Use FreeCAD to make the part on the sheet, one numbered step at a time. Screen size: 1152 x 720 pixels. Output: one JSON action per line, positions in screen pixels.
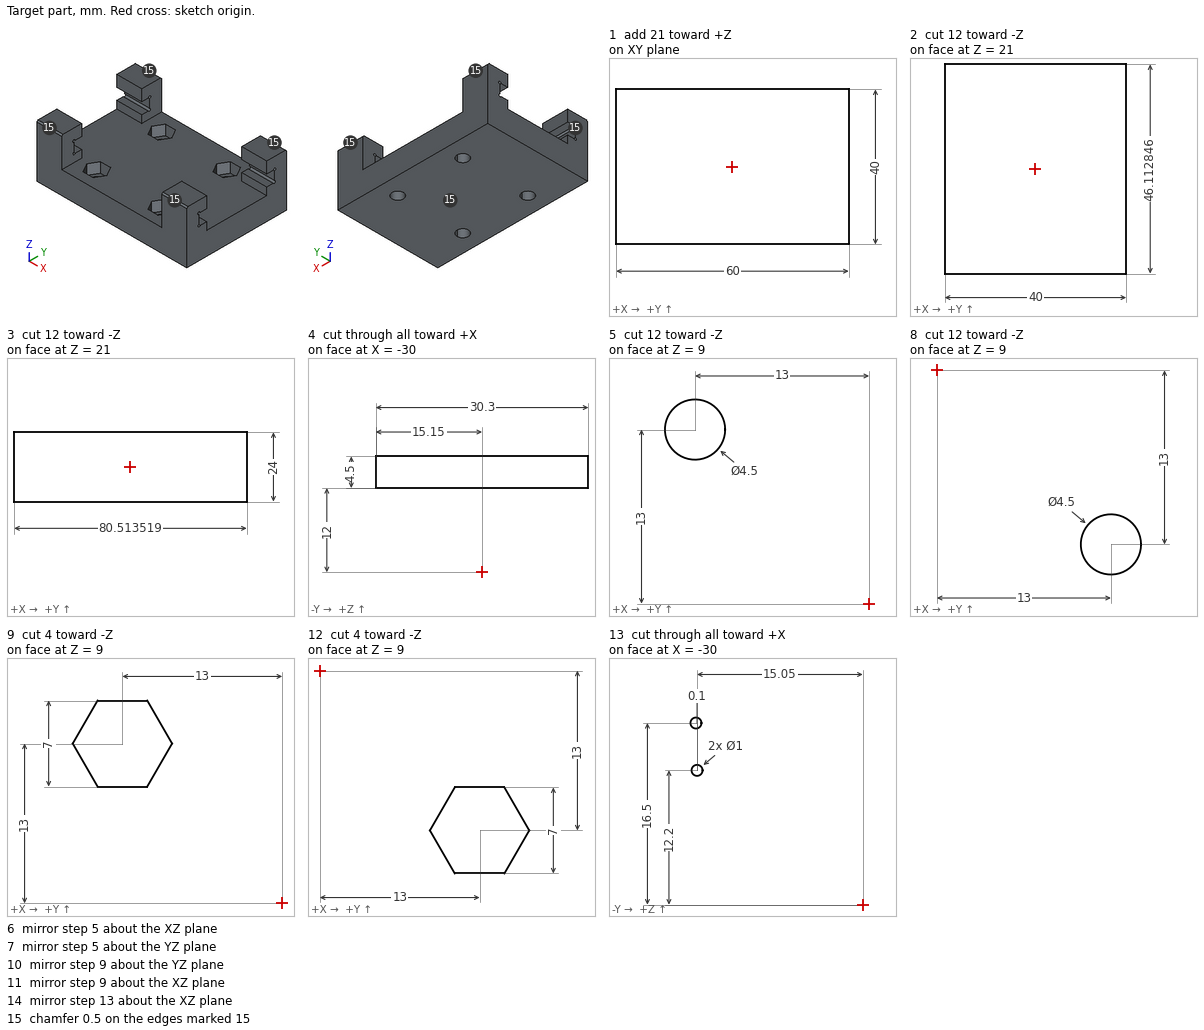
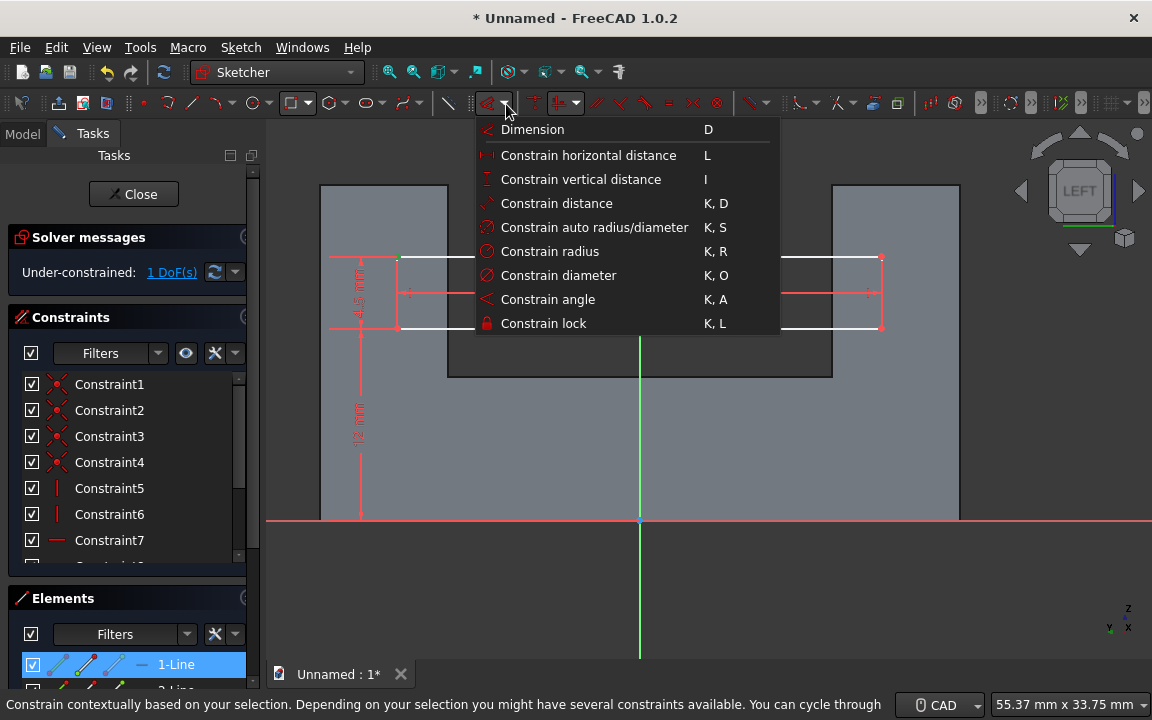
{"action": "left_click", "coordinate": [628, 155]}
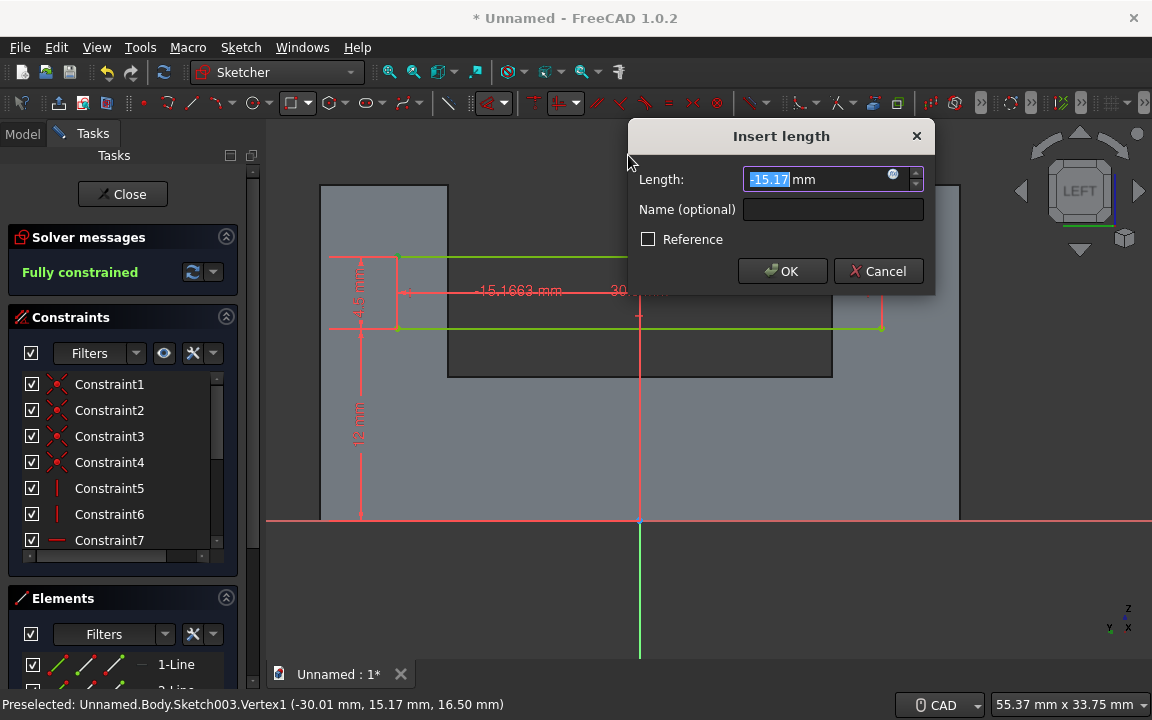
{"action": "type", "text": "-15.15"}
{"action": "key", "text": "Return"}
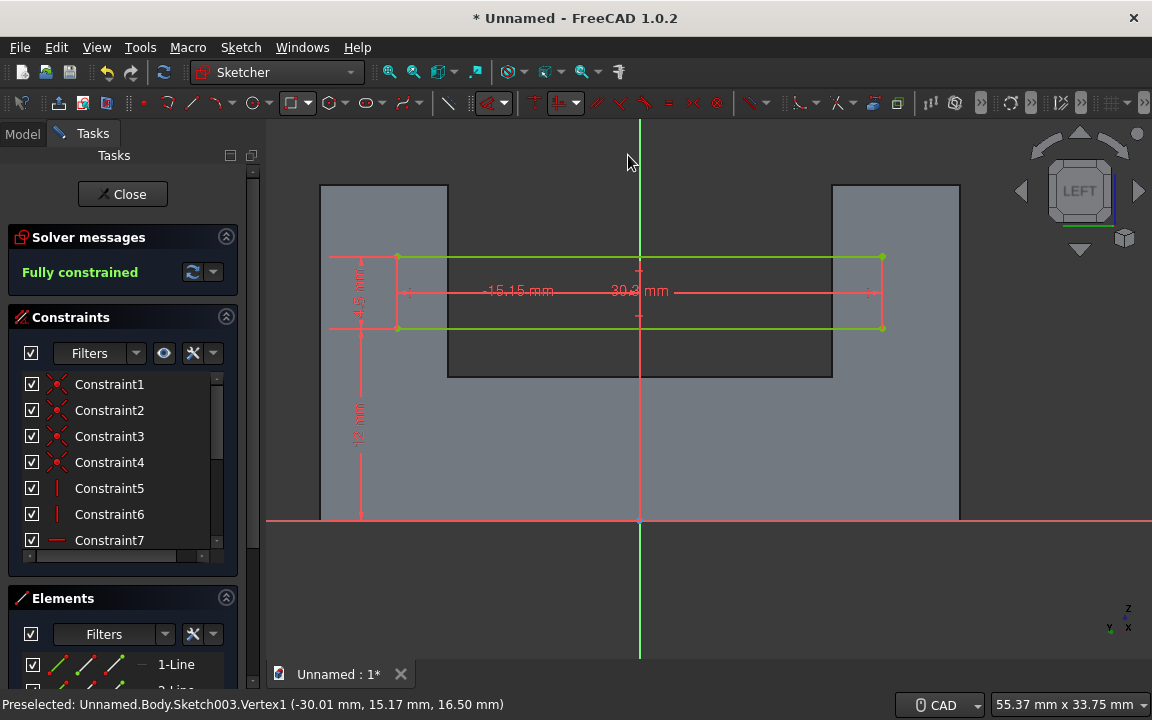
{"action": "left_click", "coordinate": [123, 194]}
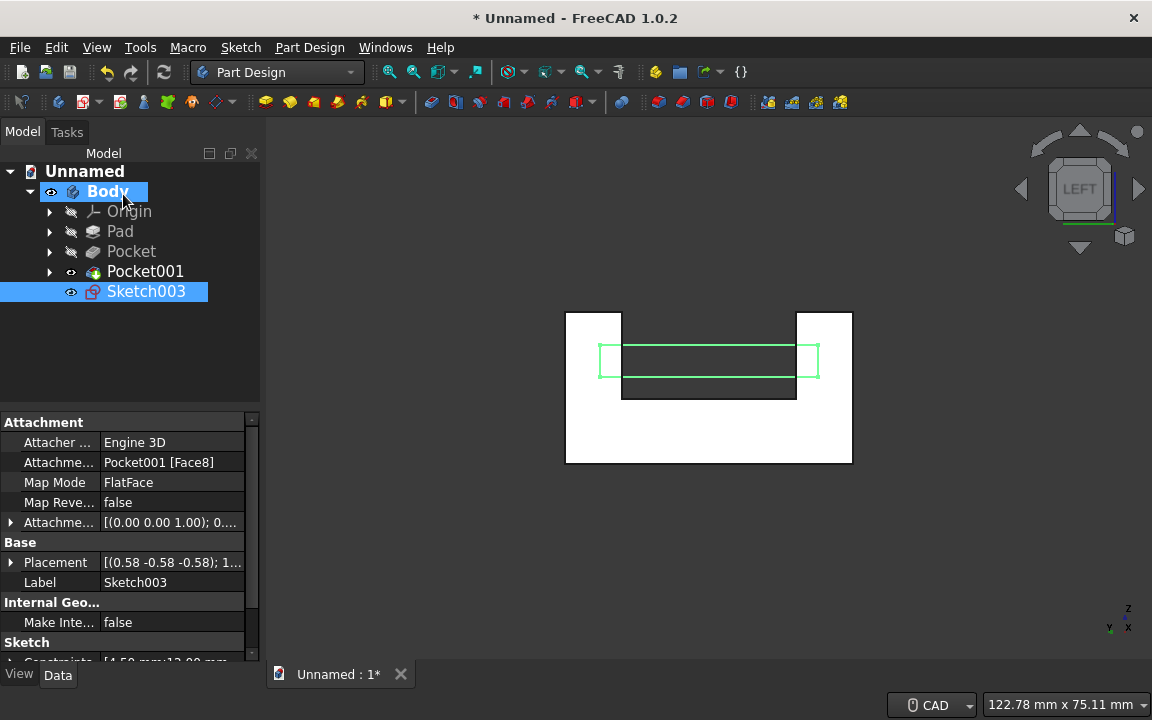
{"action": "left_click", "coordinate": [432, 102]}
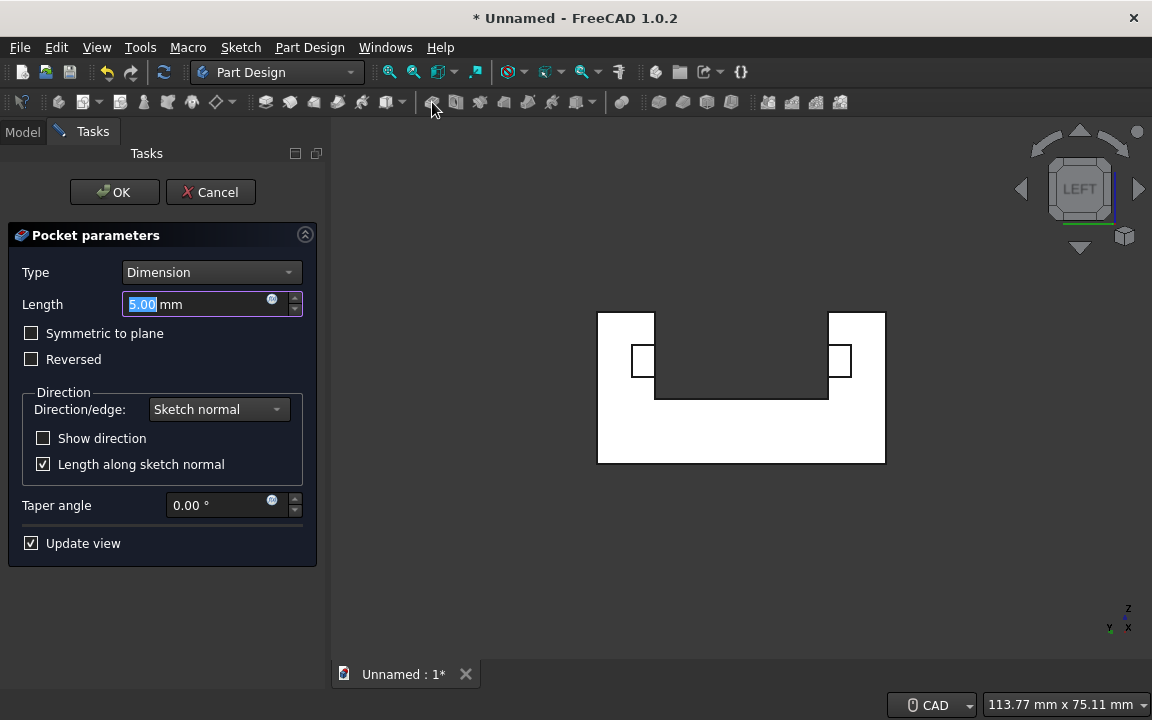
{"action": "left_click", "coordinate": [212, 272]}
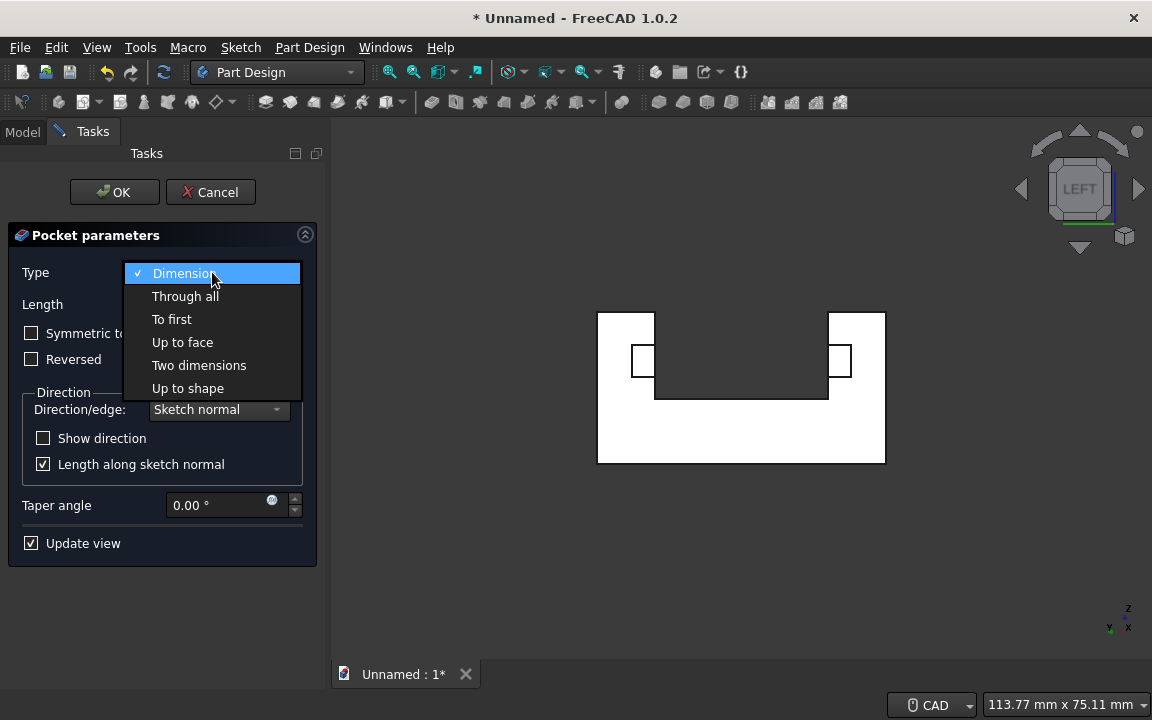
{"action": "left_click", "coordinate": [212, 296]}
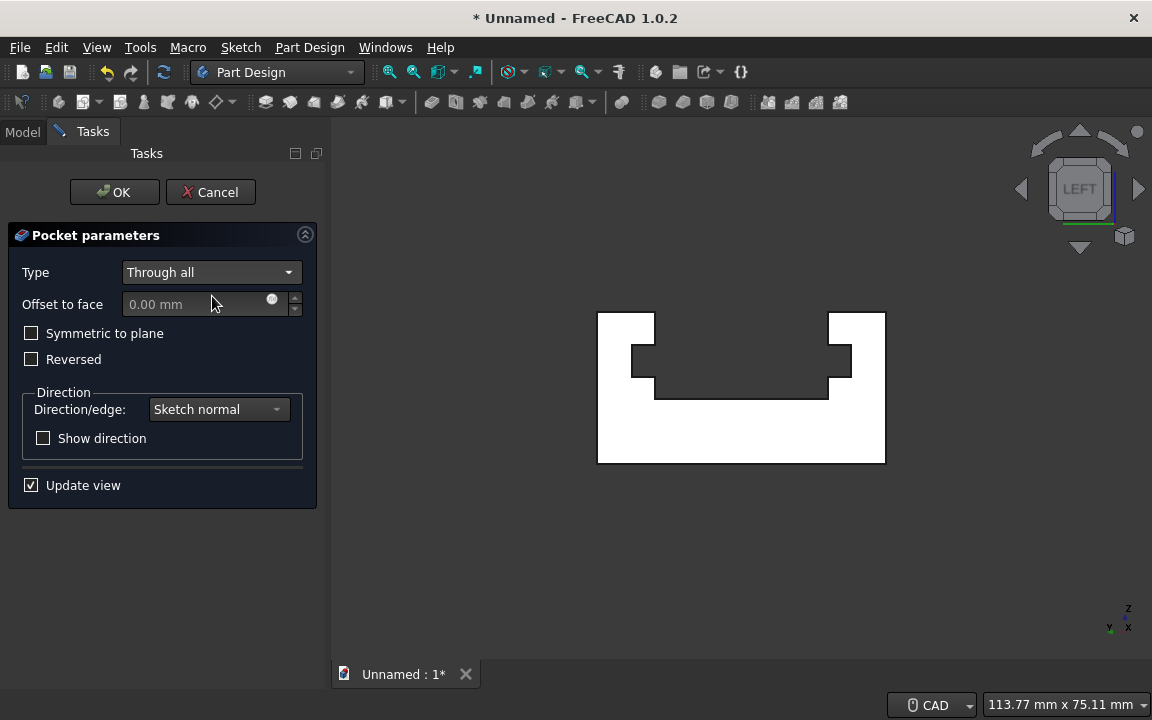
{"action": "left_click", "coordinate": [115, 192]}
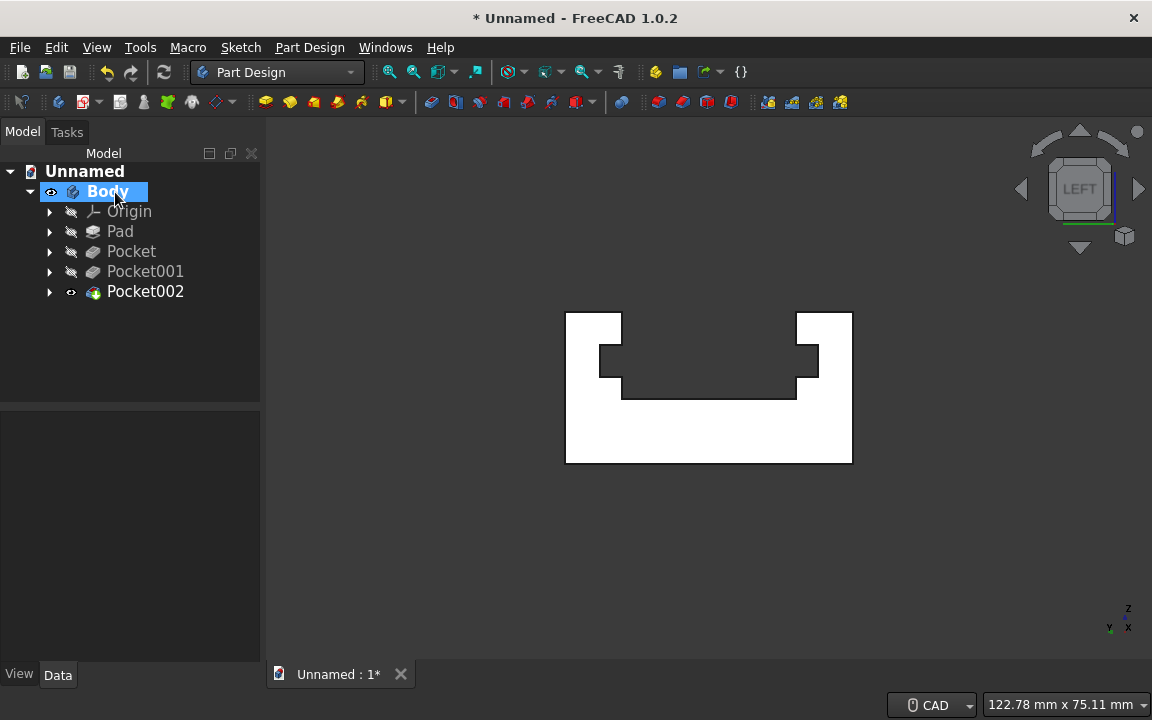
{"action": "left_click", "coordinate": [390, 72]}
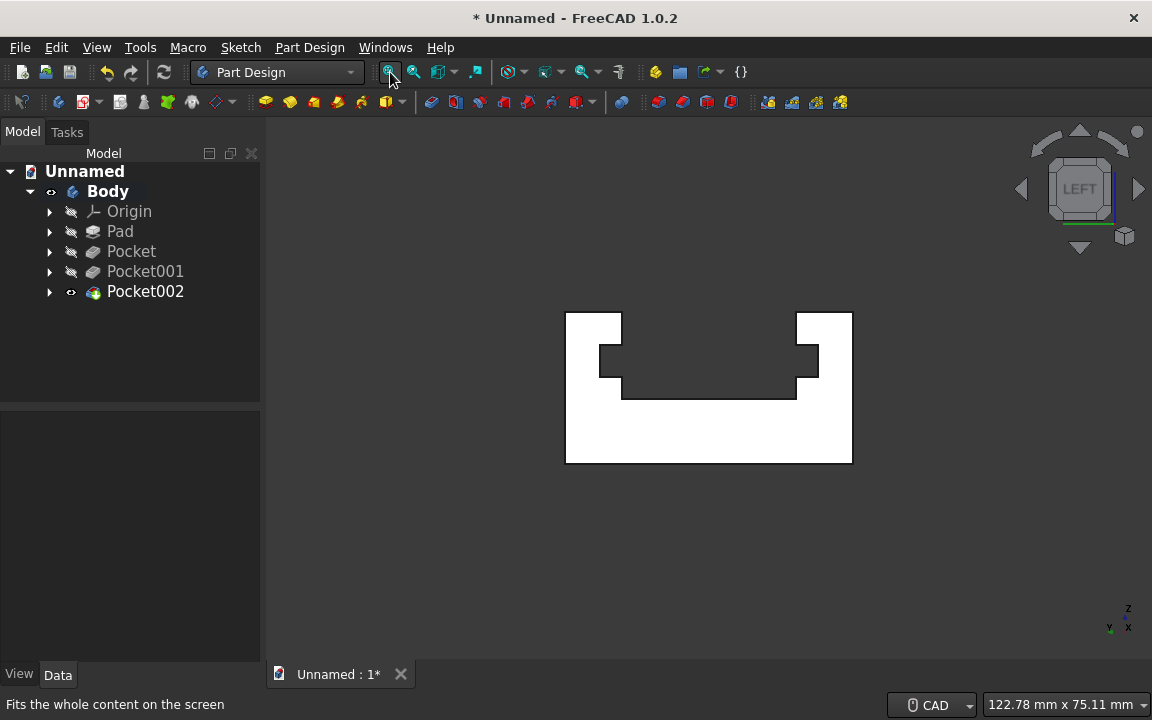
{"action": "key", "text": "0"}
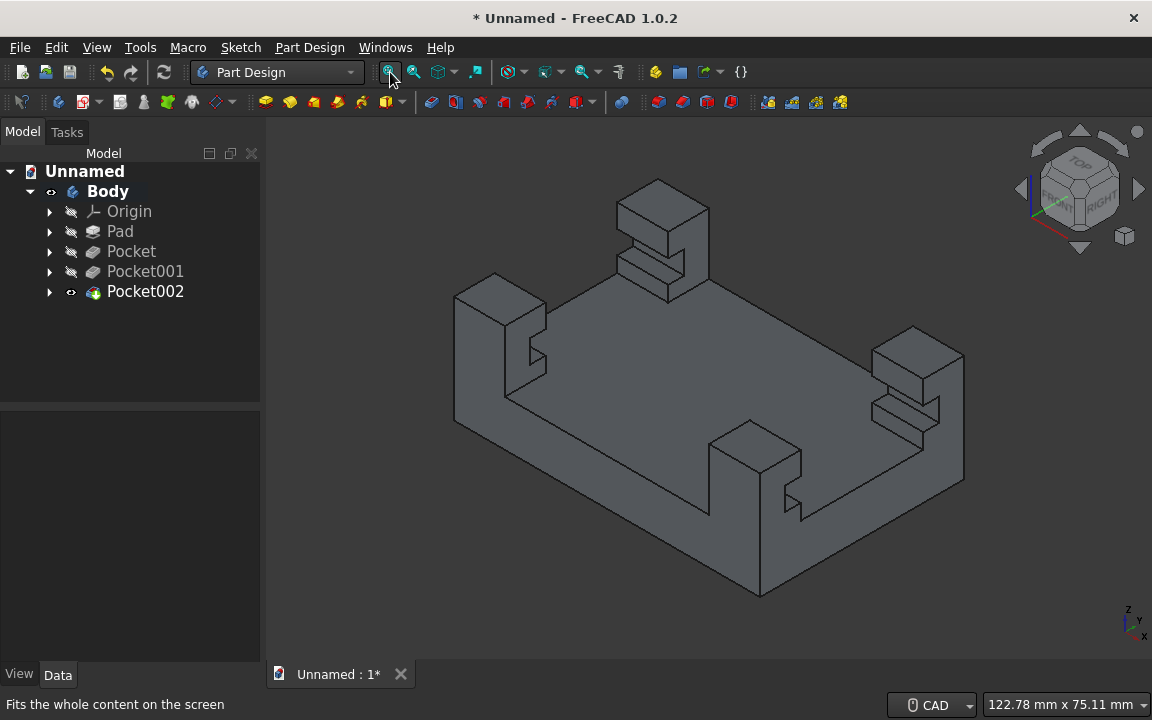
{"action": "left_click", "coordinate": [709, 396]}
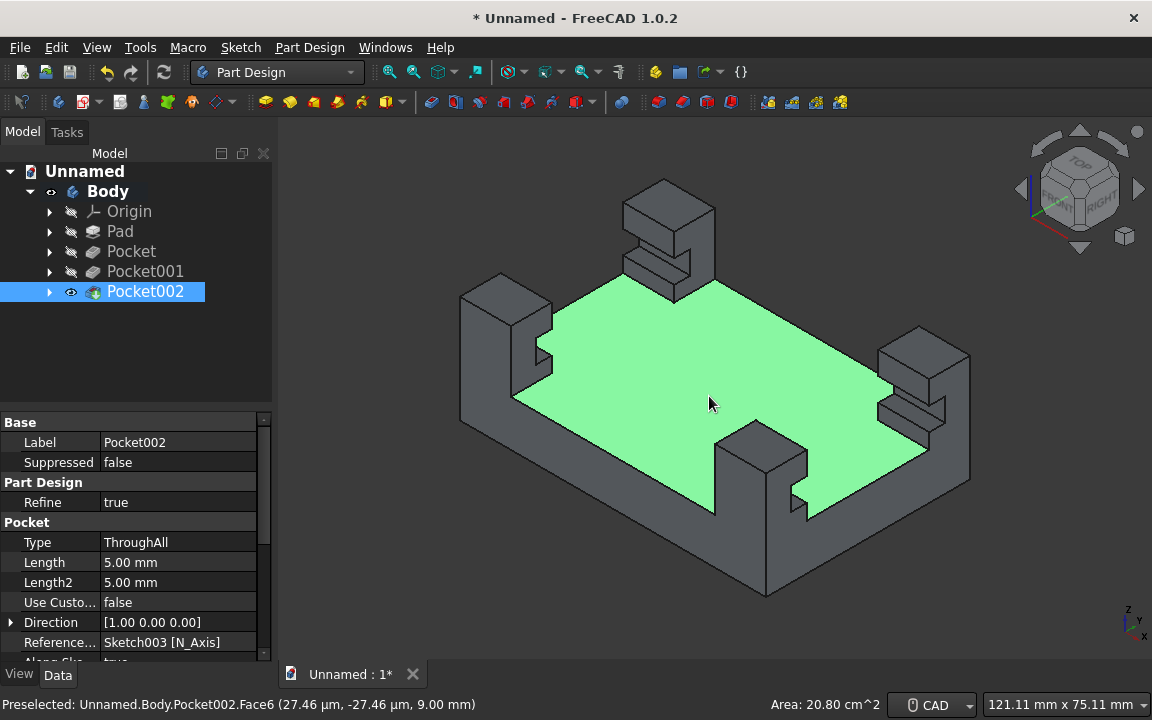
{"action": "left_click", "coordinate": [84, 102]}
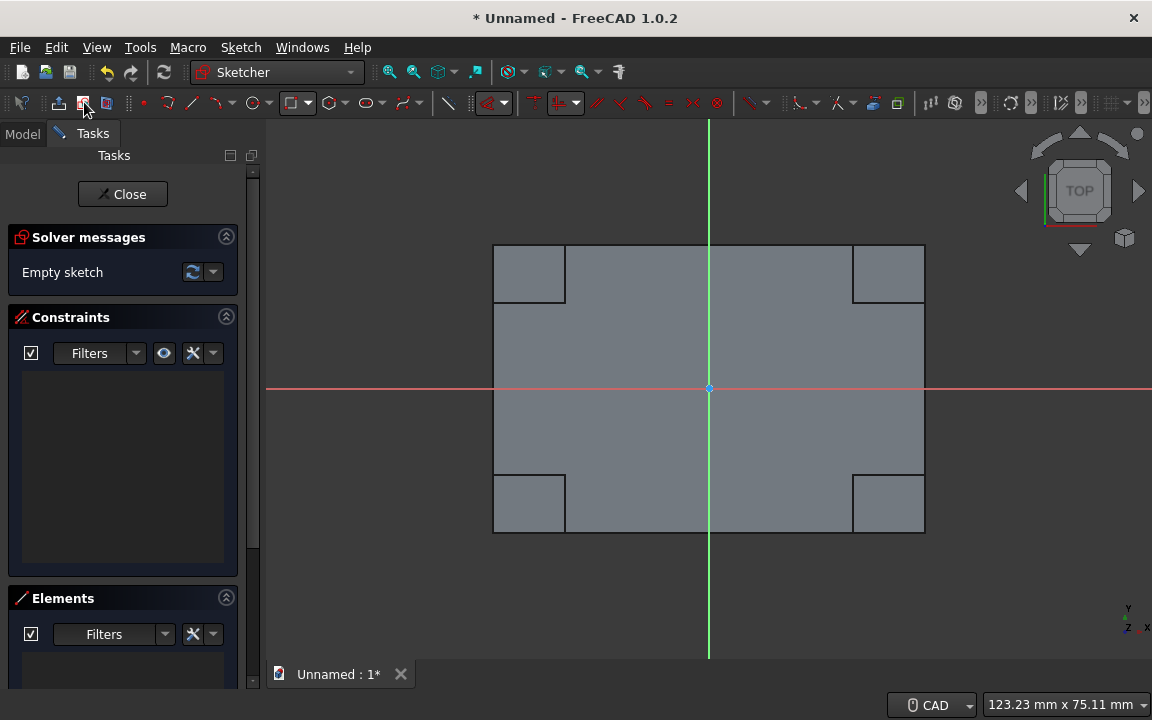
{"action": "scroll", "coordinate": [613, 286], "scroll_direction": "up", "scroll_amount": 12}